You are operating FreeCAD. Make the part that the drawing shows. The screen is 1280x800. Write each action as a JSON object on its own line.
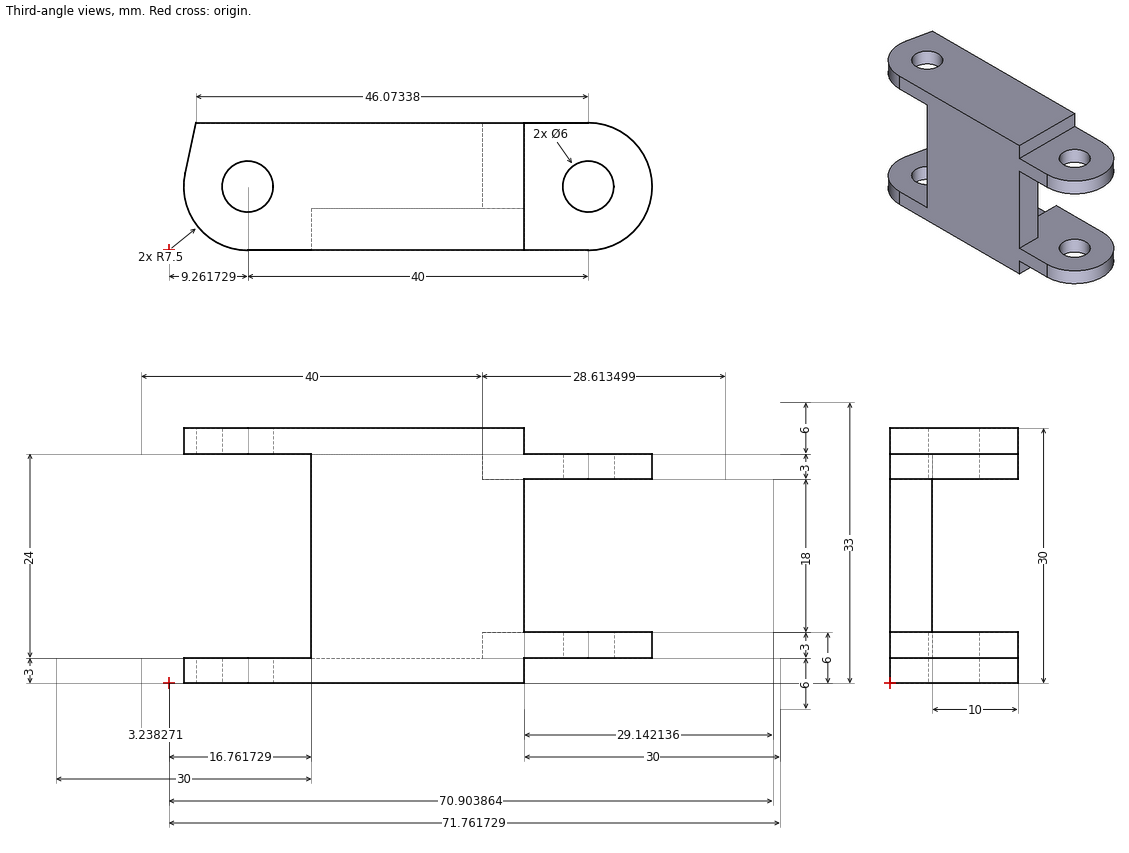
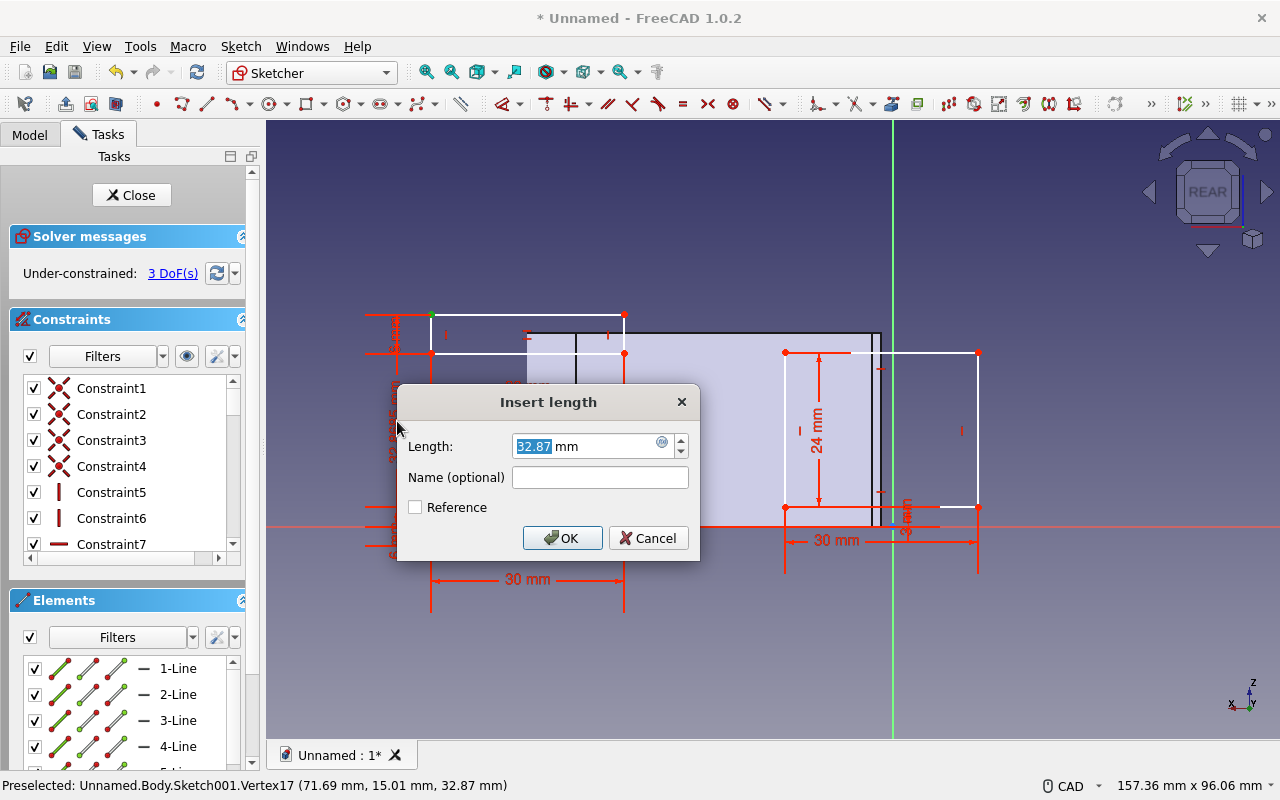
{"action": "type", "text": "33"}
{"action": "key", "text": "Return"}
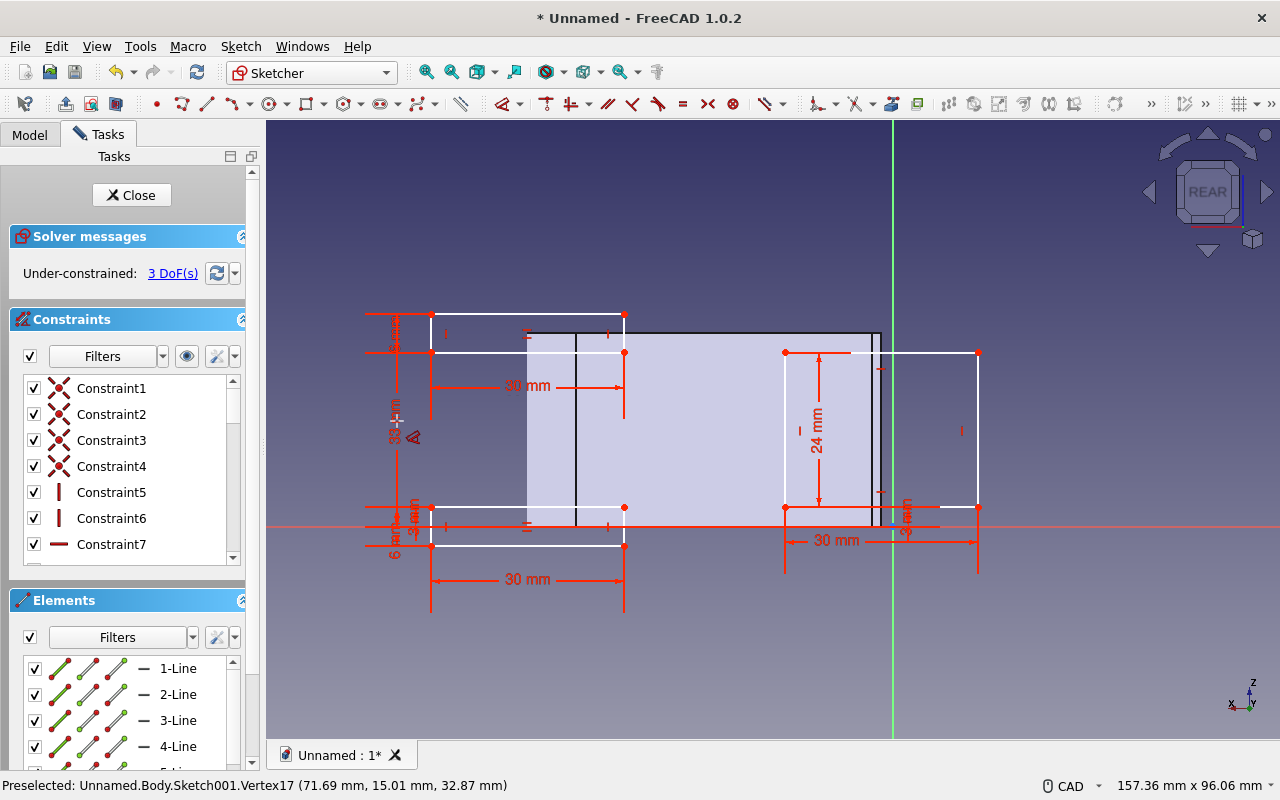
{"action": "left_click", "coordinate": [785, 353]}
{"action": "left_click", "coordinate": [839, 319]}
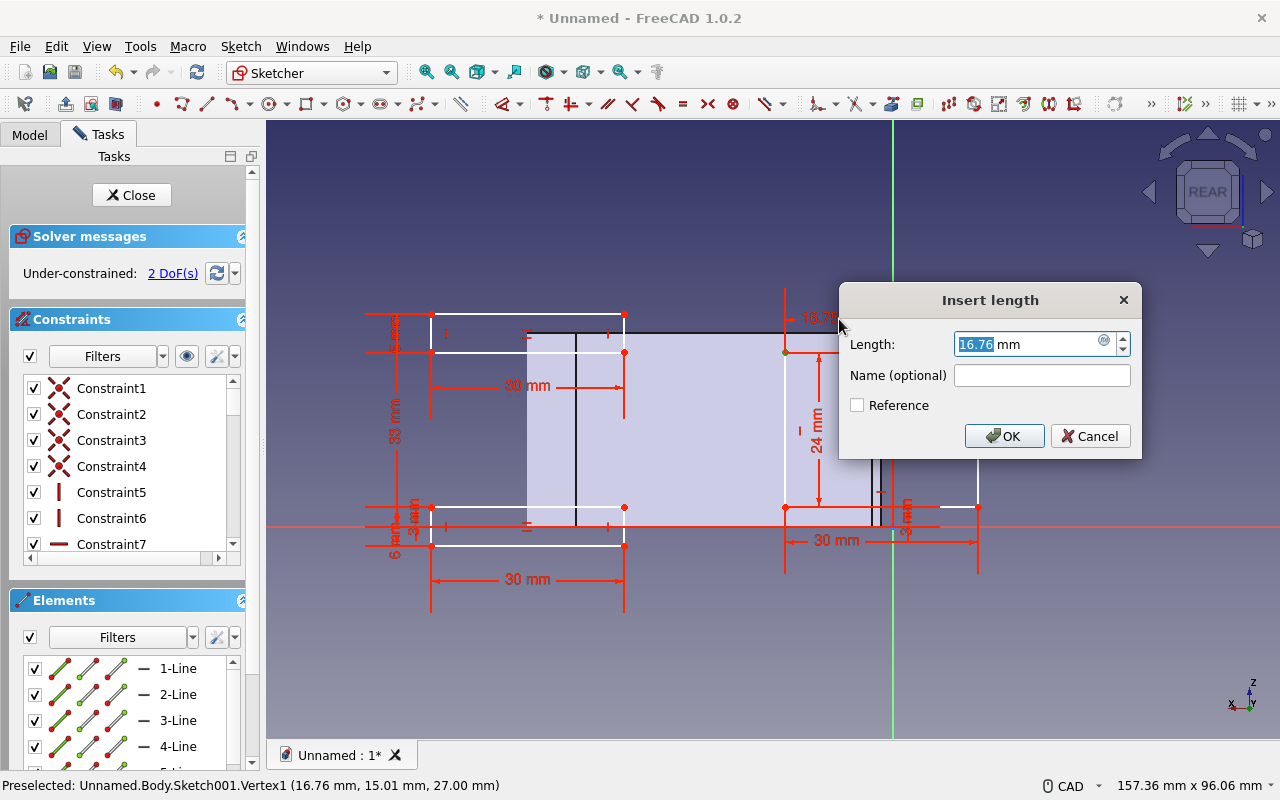
{"action": "type", "text": "16.761729"}
{"action": "key", "text": "Return"}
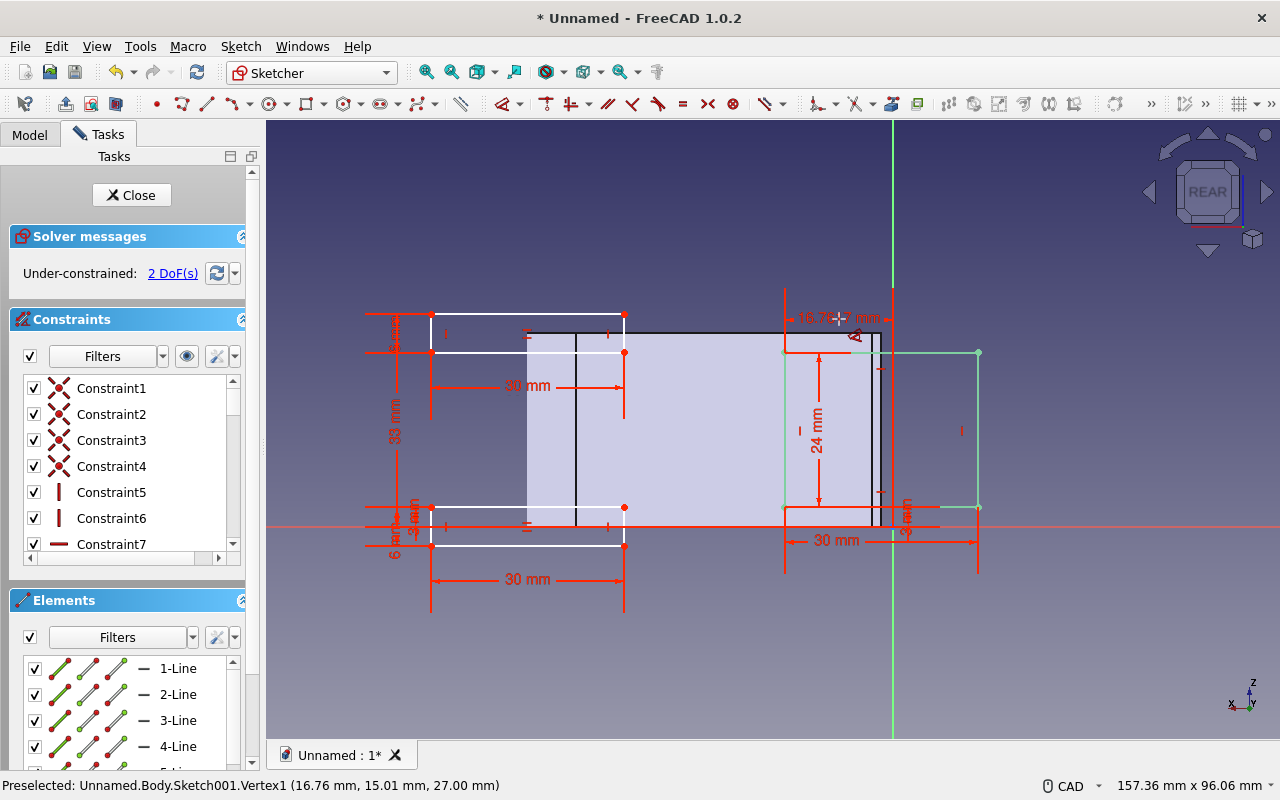
{"action": "left_click", "coordinate": [431, 507]}
{"action": "left_click", "coordinate": [662, 561]}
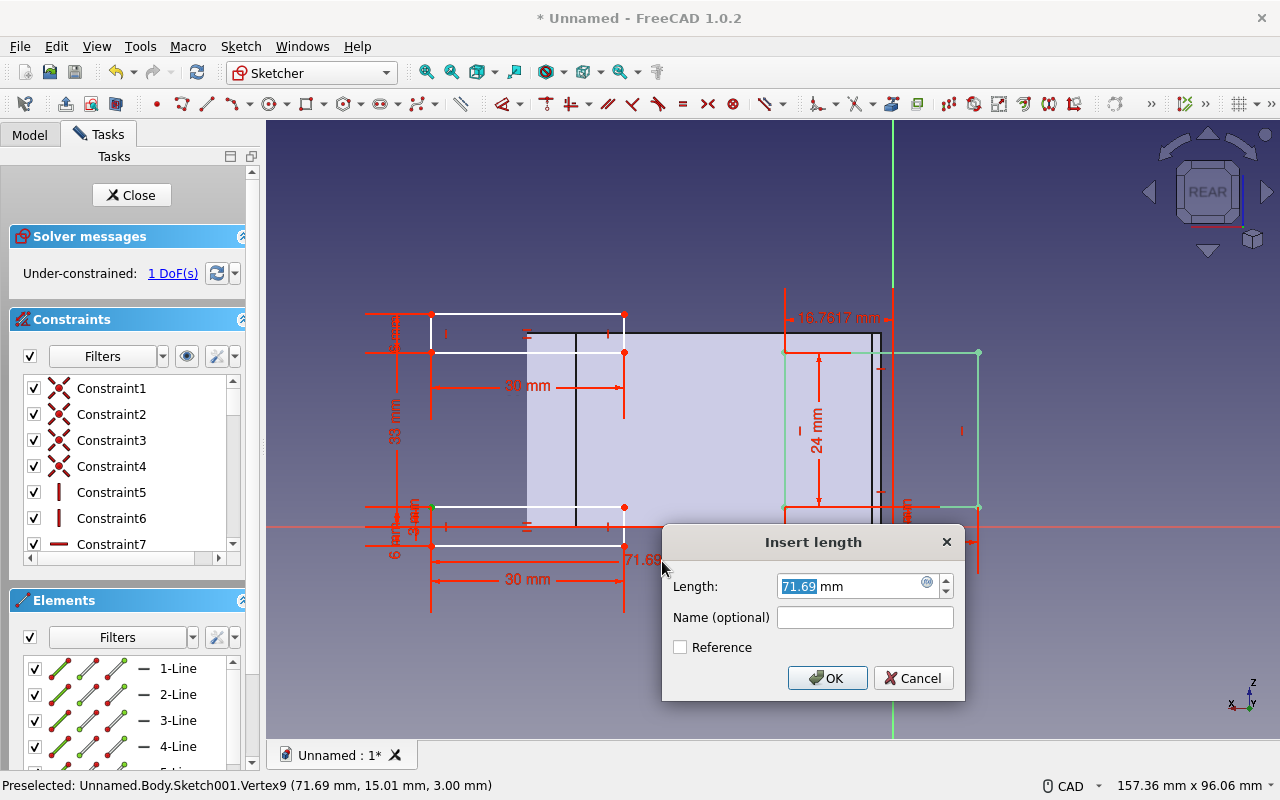
{"action": "type", "text": "71.761729"}
{"action": "key", "text": "Return"}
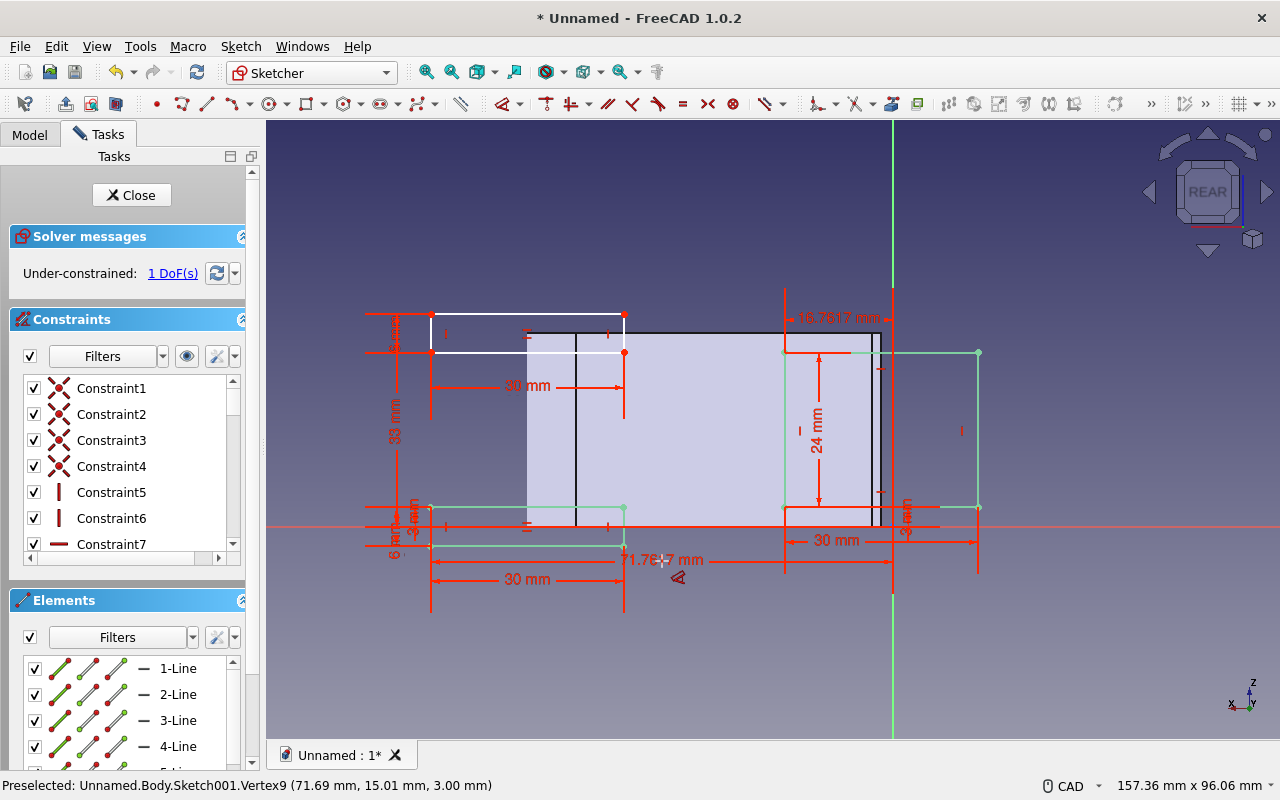
{"action": "left_click", "coordinate": [431, 314]}
{"action": "left_click", "coordinate": [662, 280]}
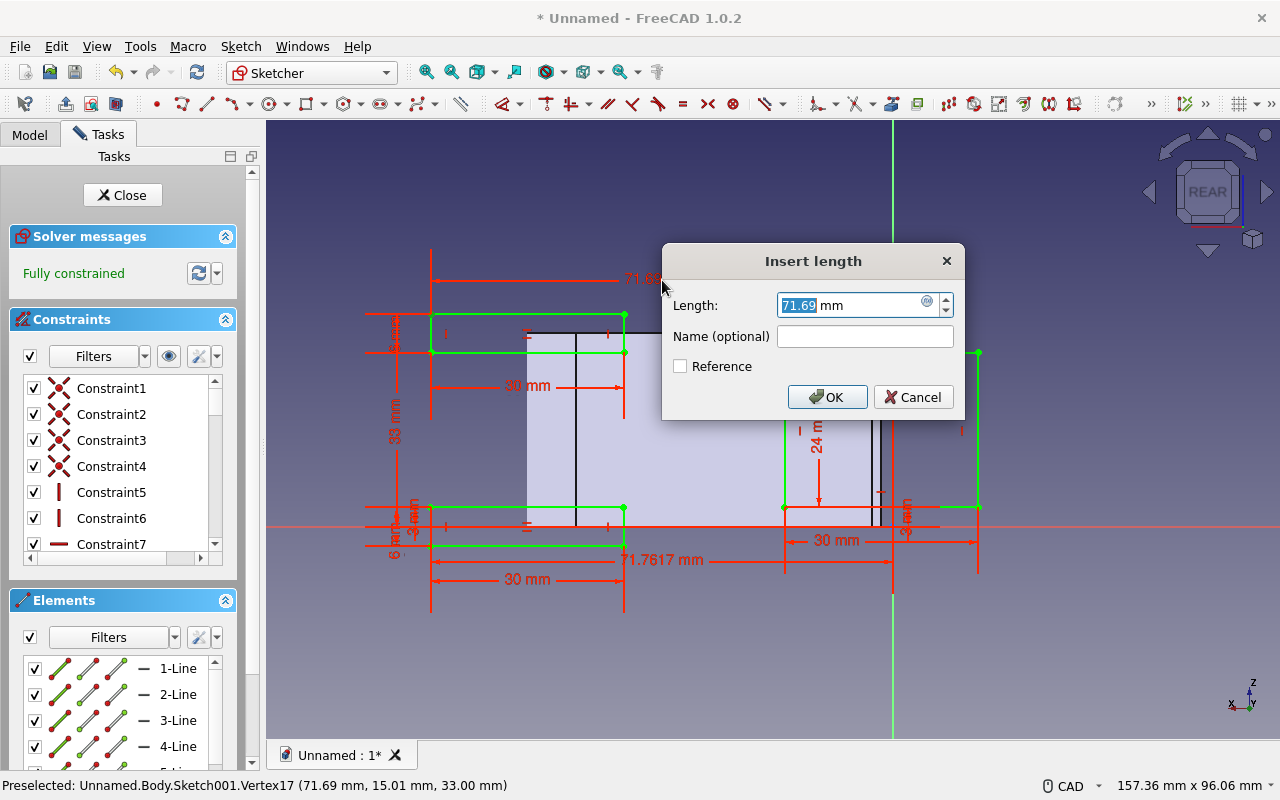
{"action": "type", "text": "71.761729"}
{"action": "key", "text": "Return"}
{"action": "key", "text": "Escape"}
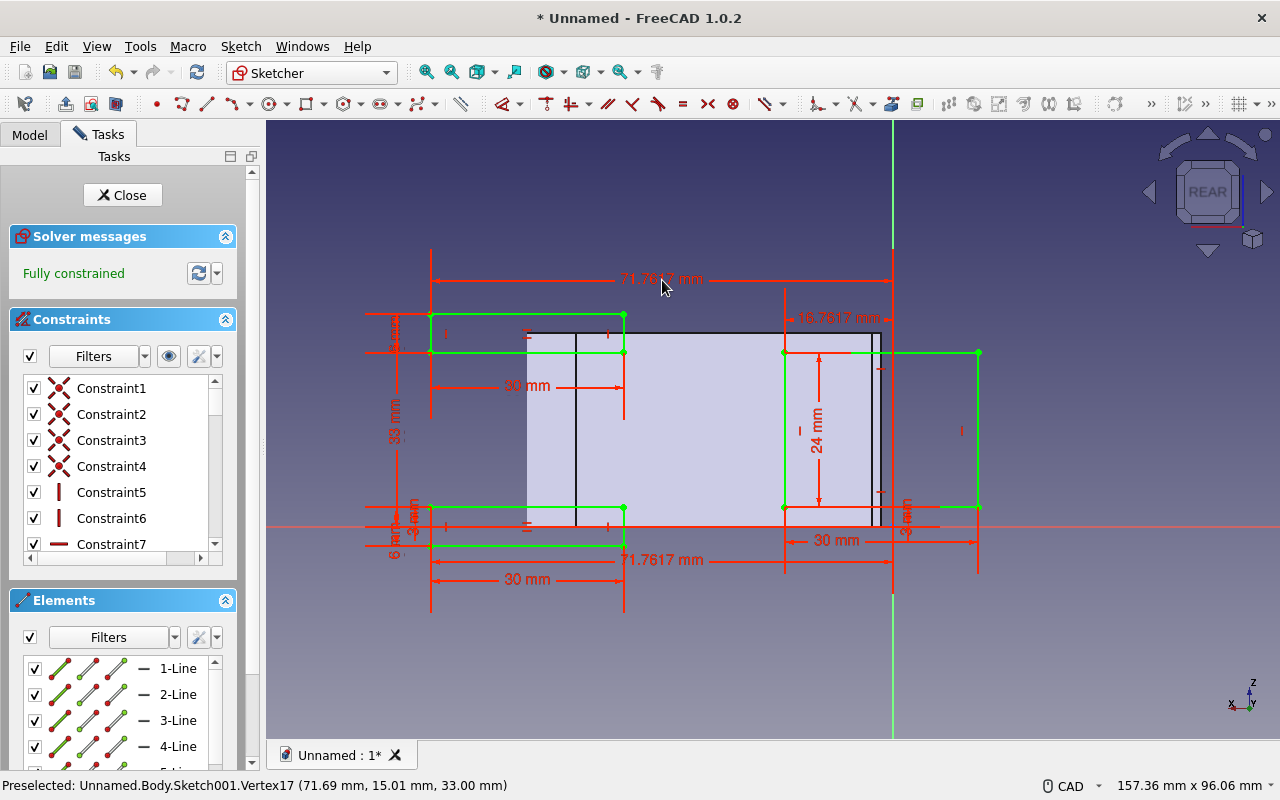
{"action": "left_click", "coordinate": [123, 195]}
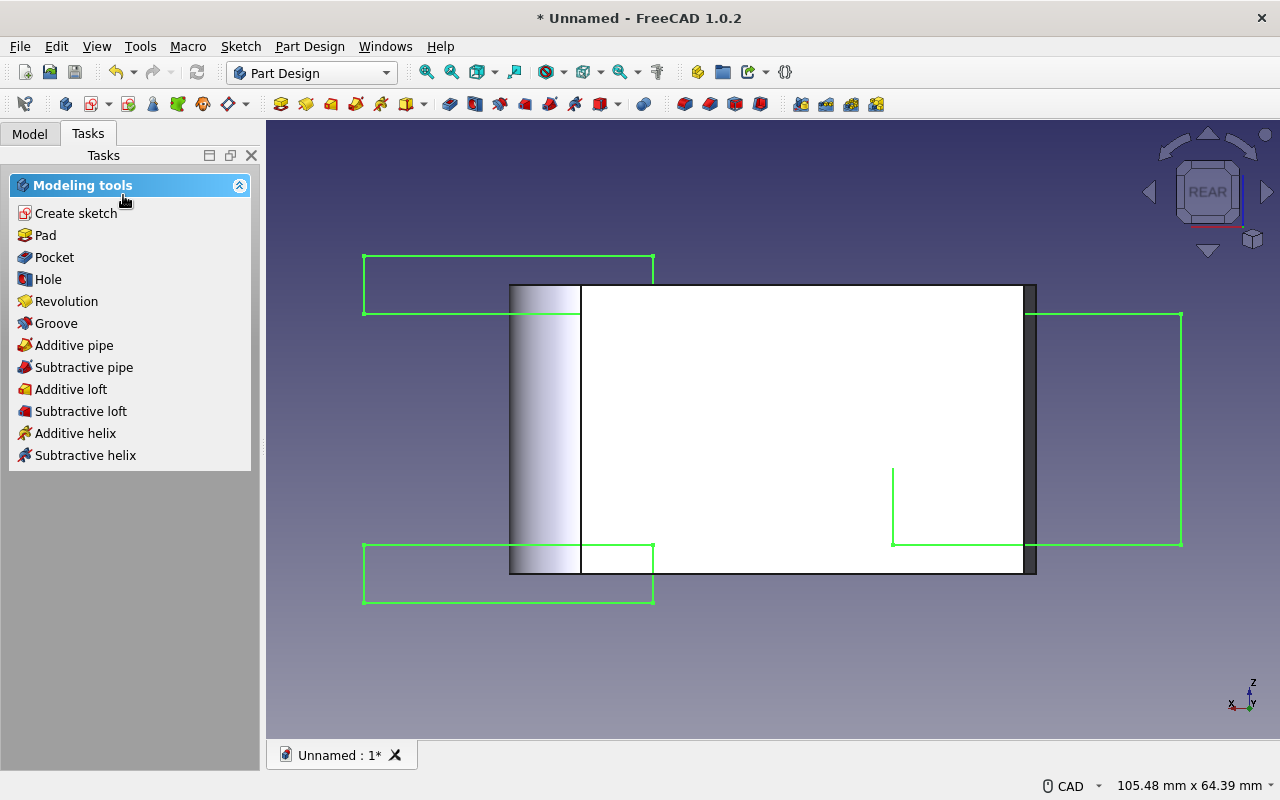
{"action": "left_click", "coordinate": [450, 104]}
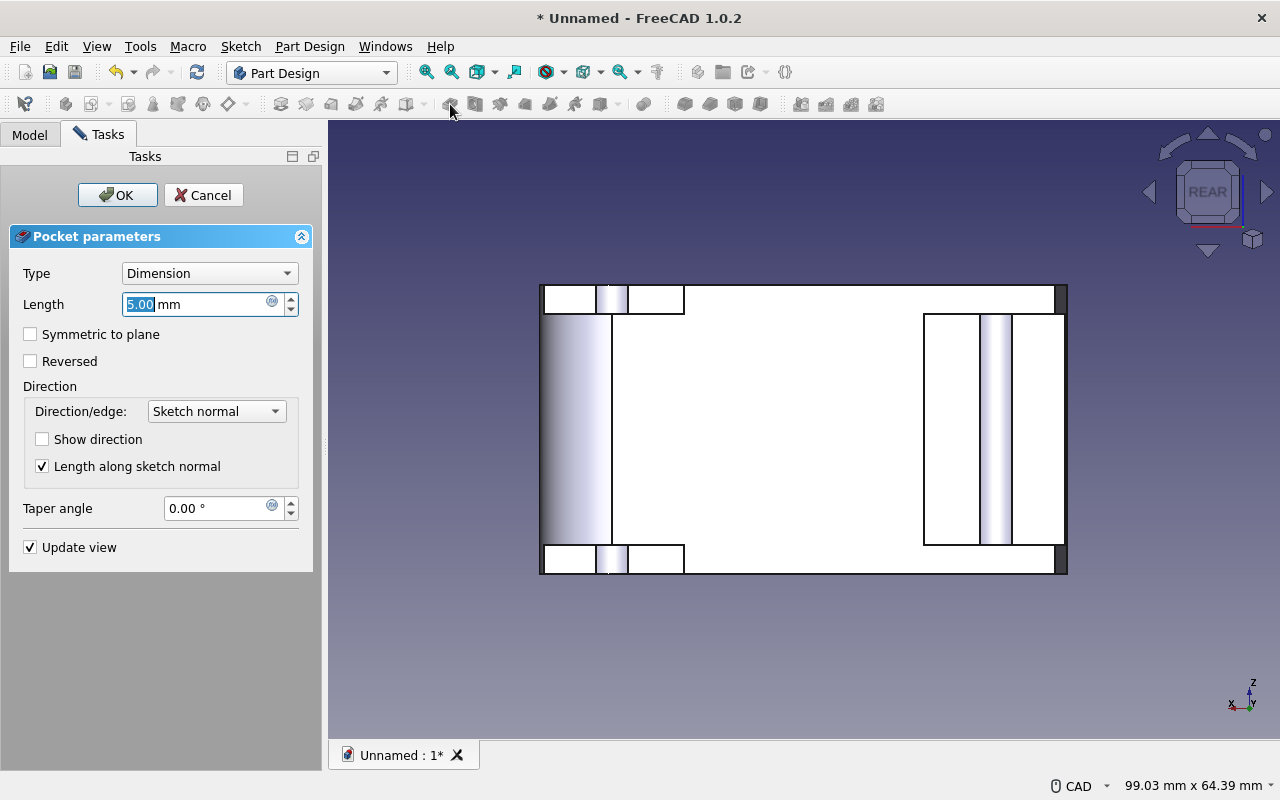
{"action": "type", "text": "30"}
{"action": "key", "text": "Tab"}